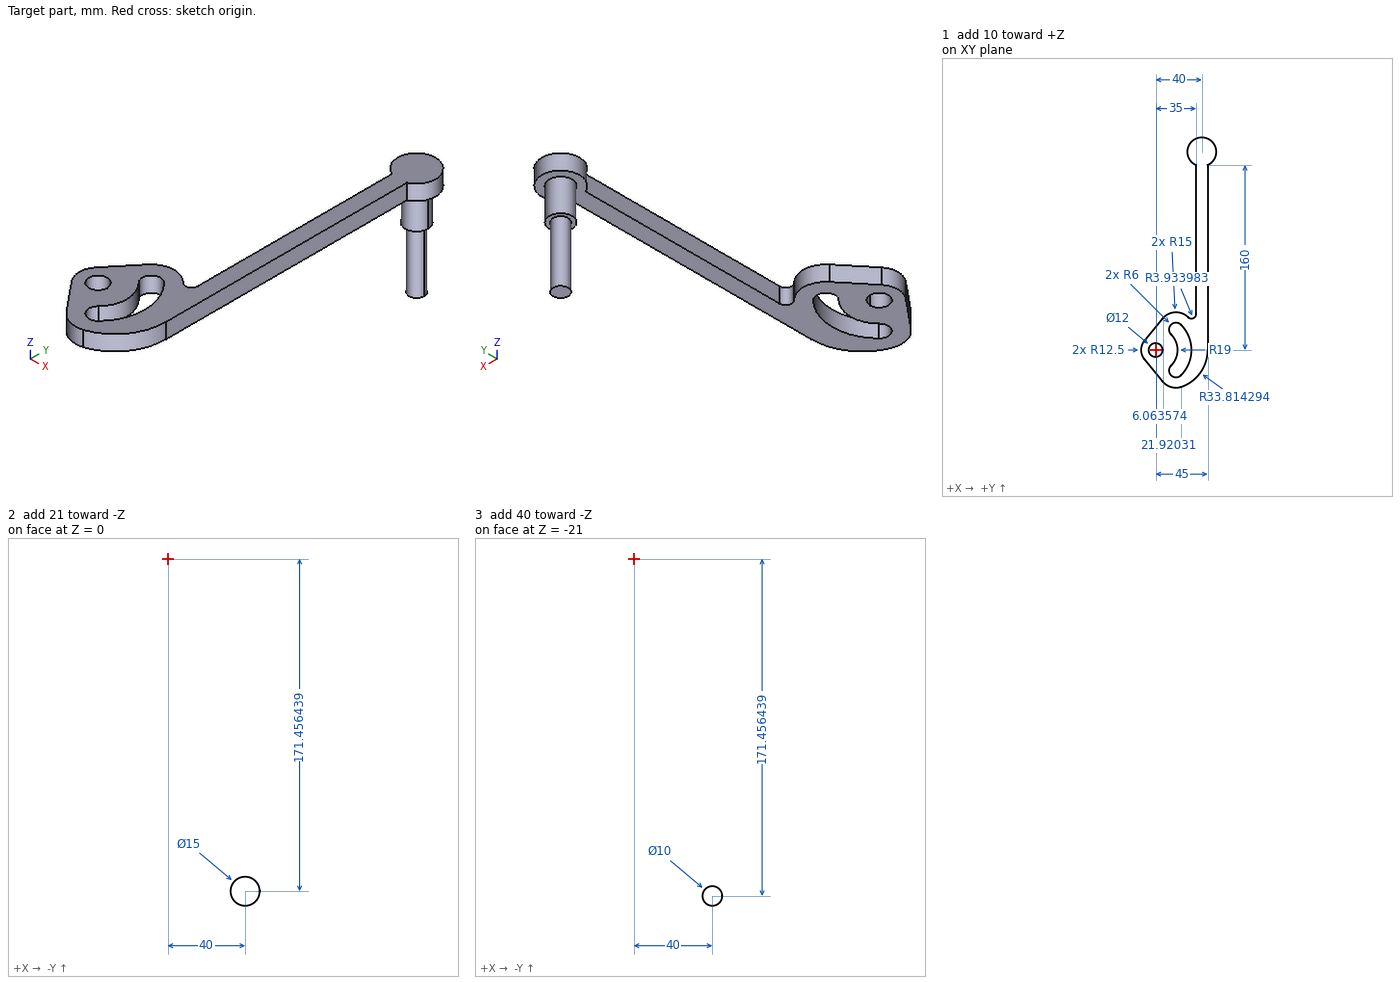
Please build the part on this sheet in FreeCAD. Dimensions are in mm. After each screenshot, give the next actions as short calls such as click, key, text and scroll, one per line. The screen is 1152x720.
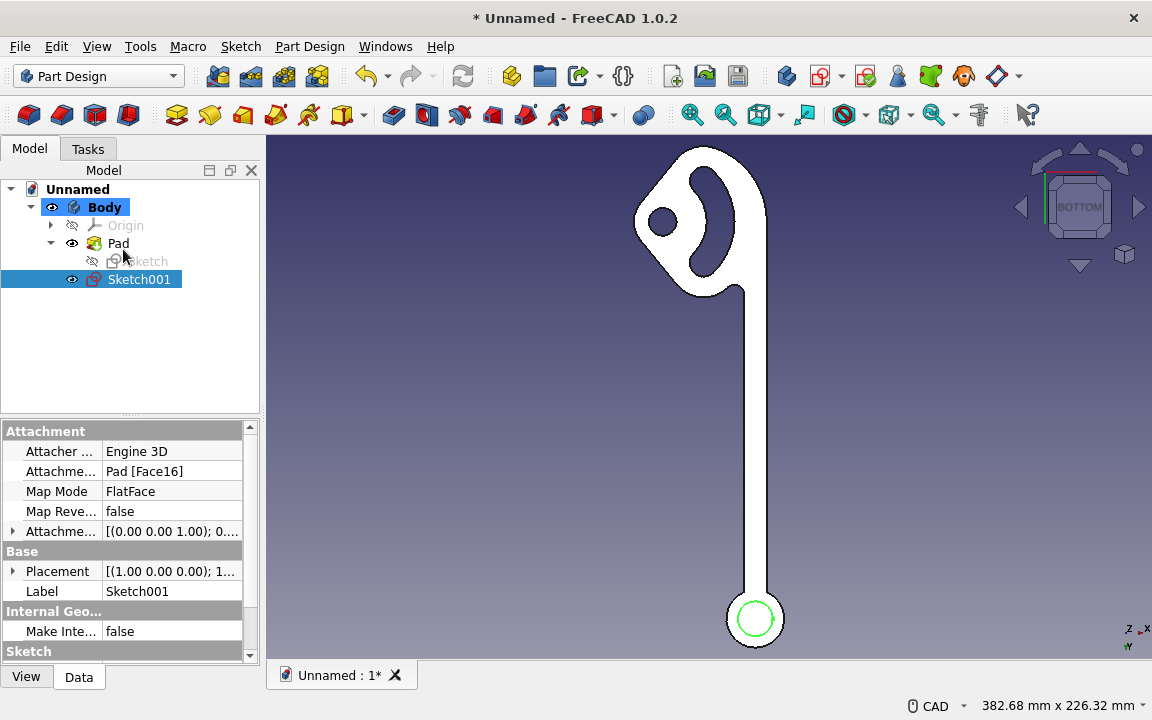
click(177, 116)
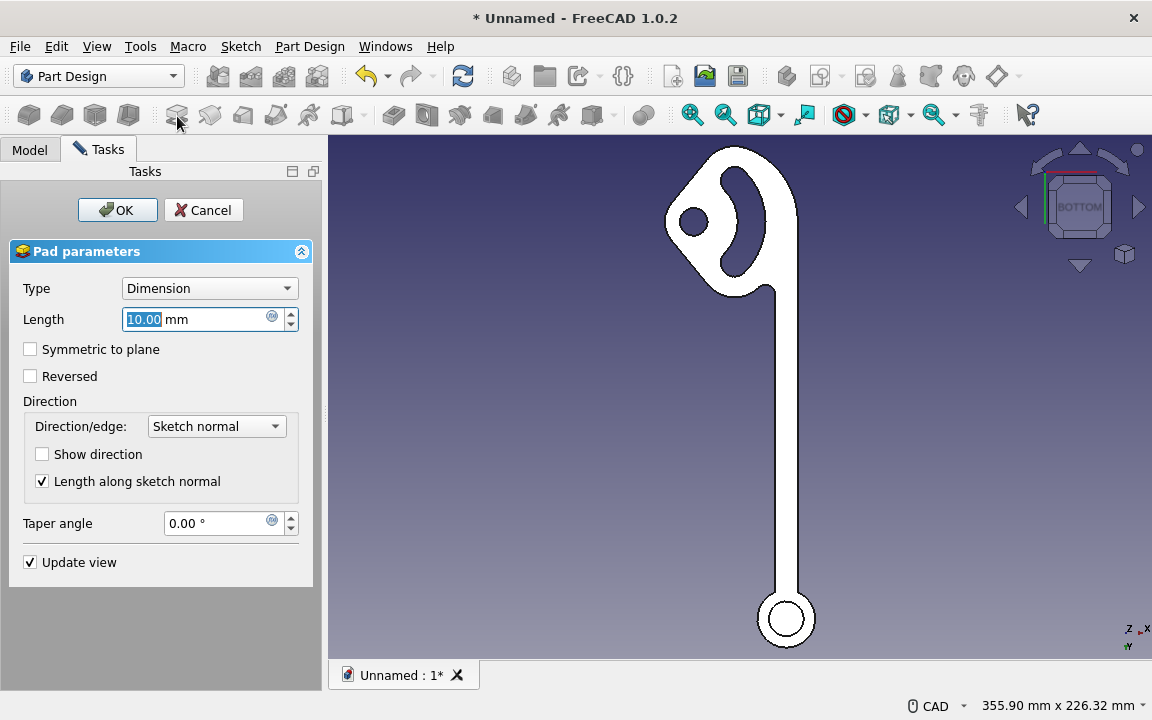
text(21)
key(Tab)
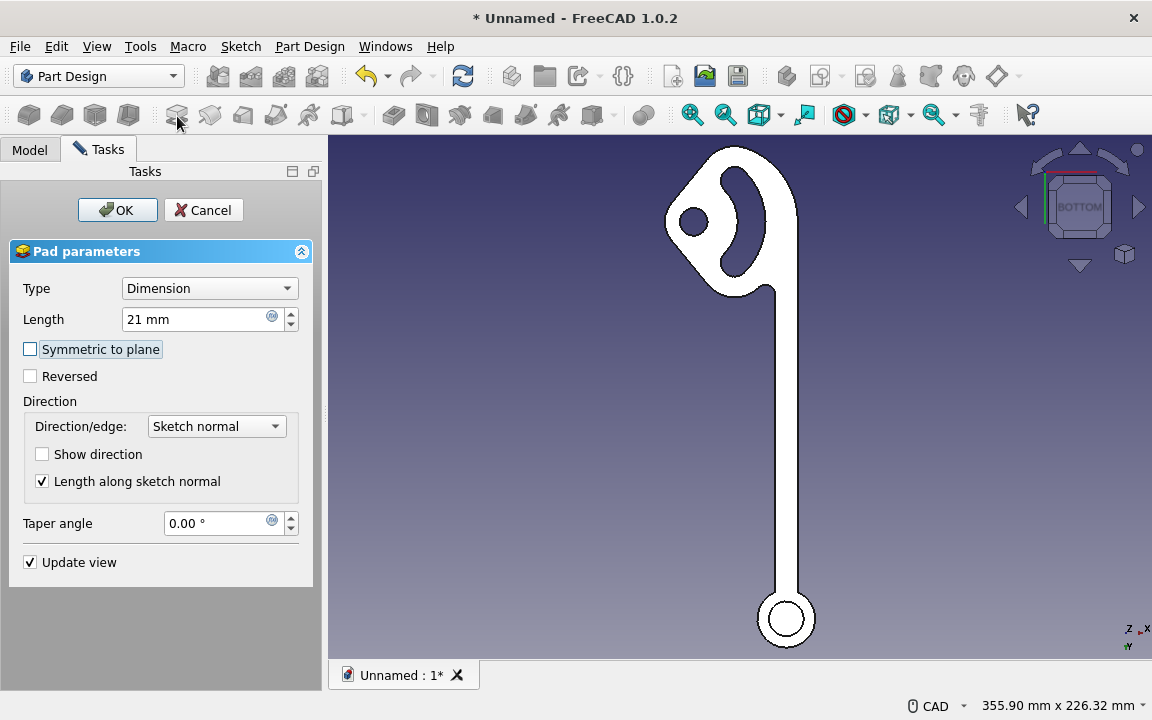
click(118, 210)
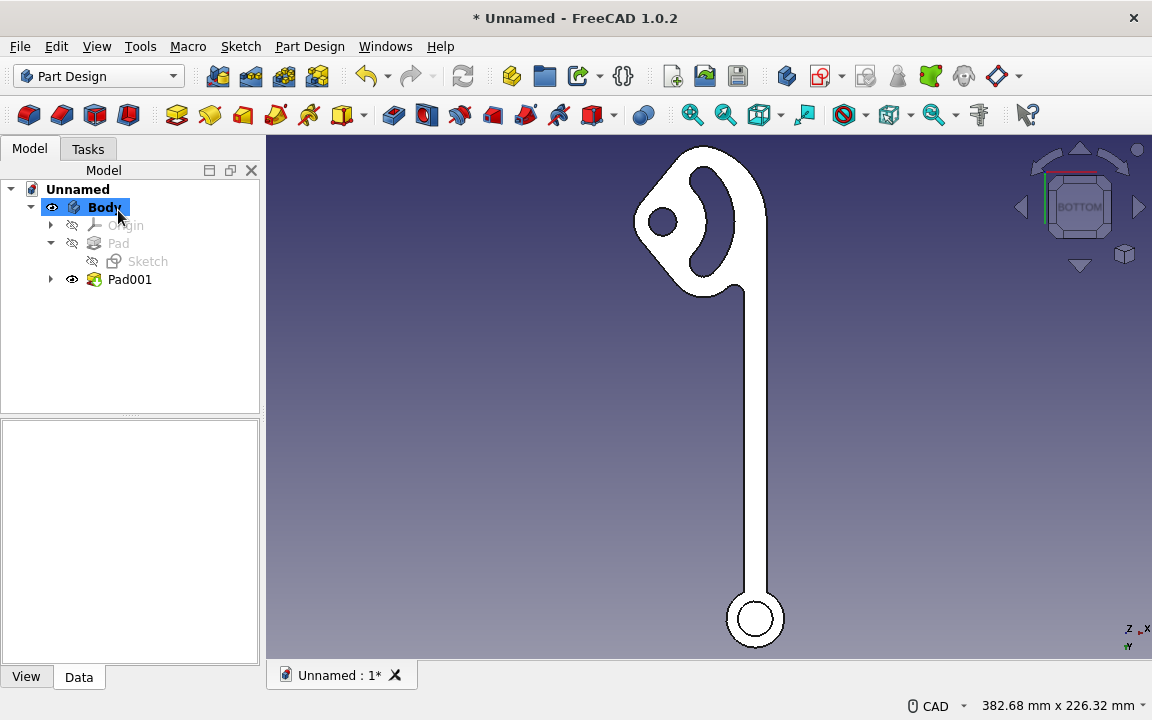
click(755, 618)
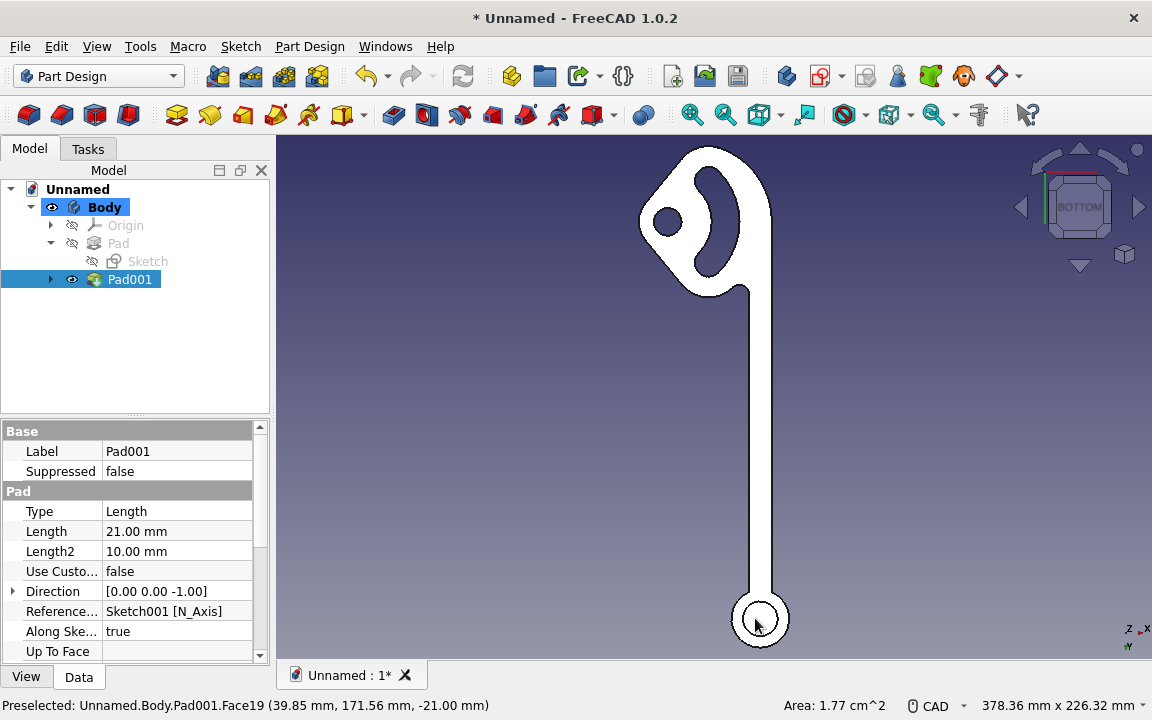
click(820, 76)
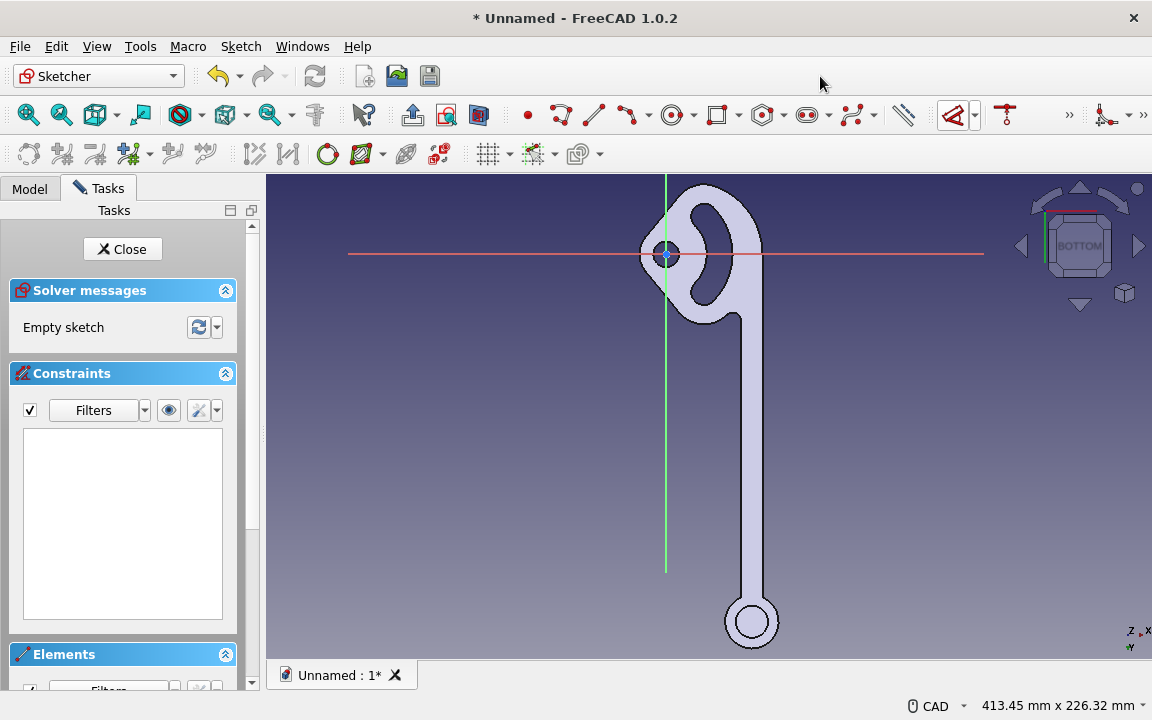
scroll(640, 416, down, 5)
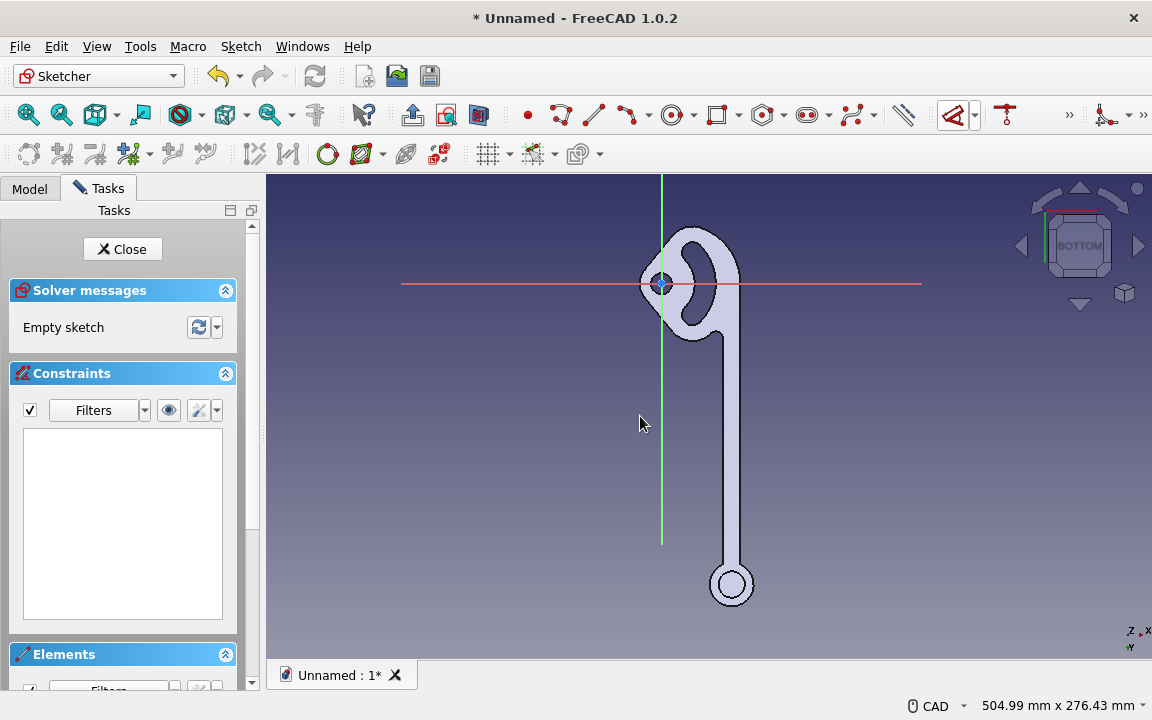
scroll(684, 496, up, 15)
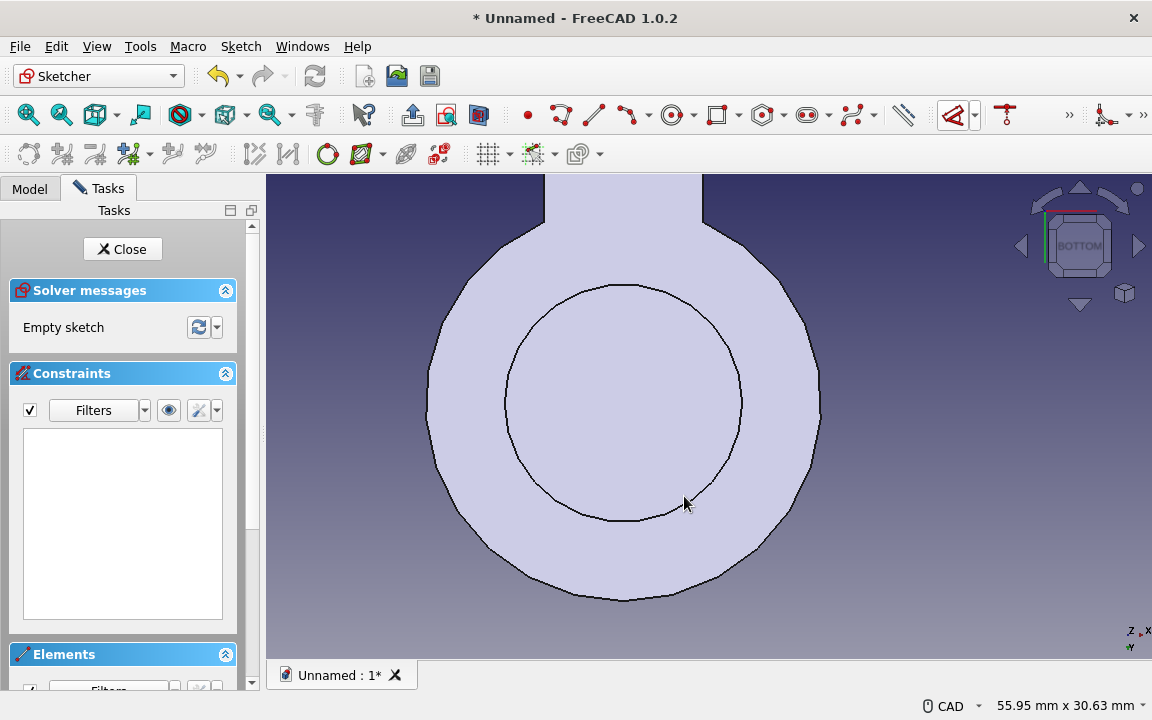
scroll(603, 387, up, 3)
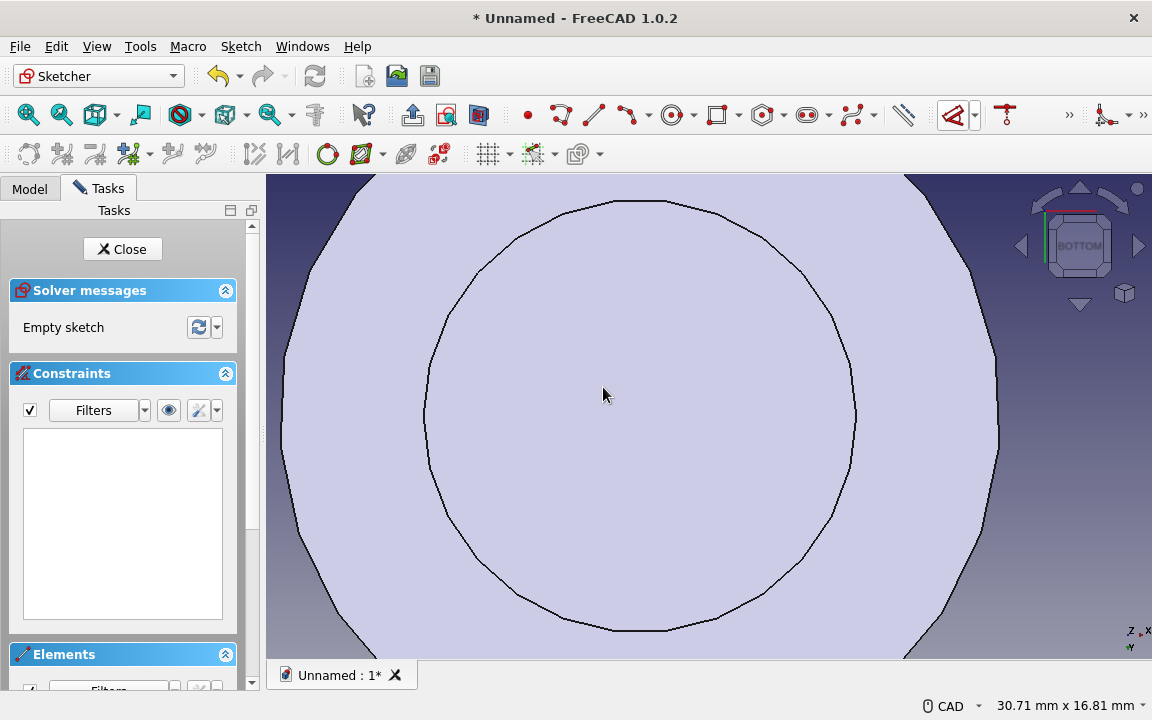
key(g)
key(c)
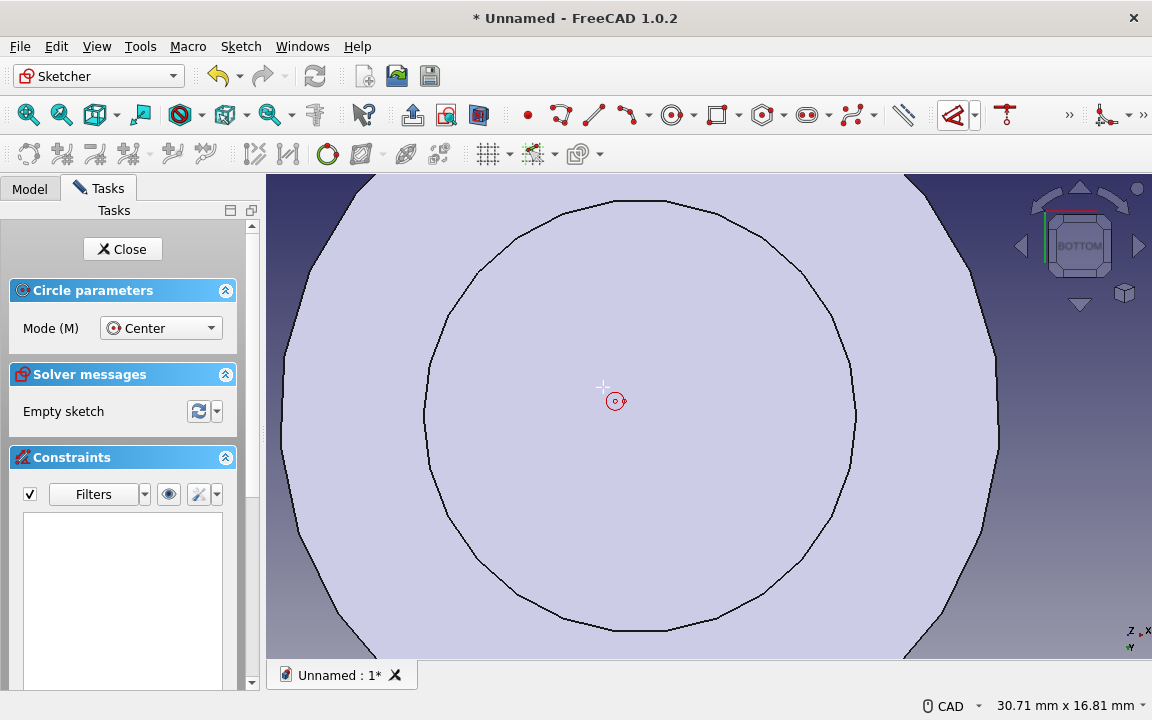
click(640, 416)
click(742, 314)
key(Escape)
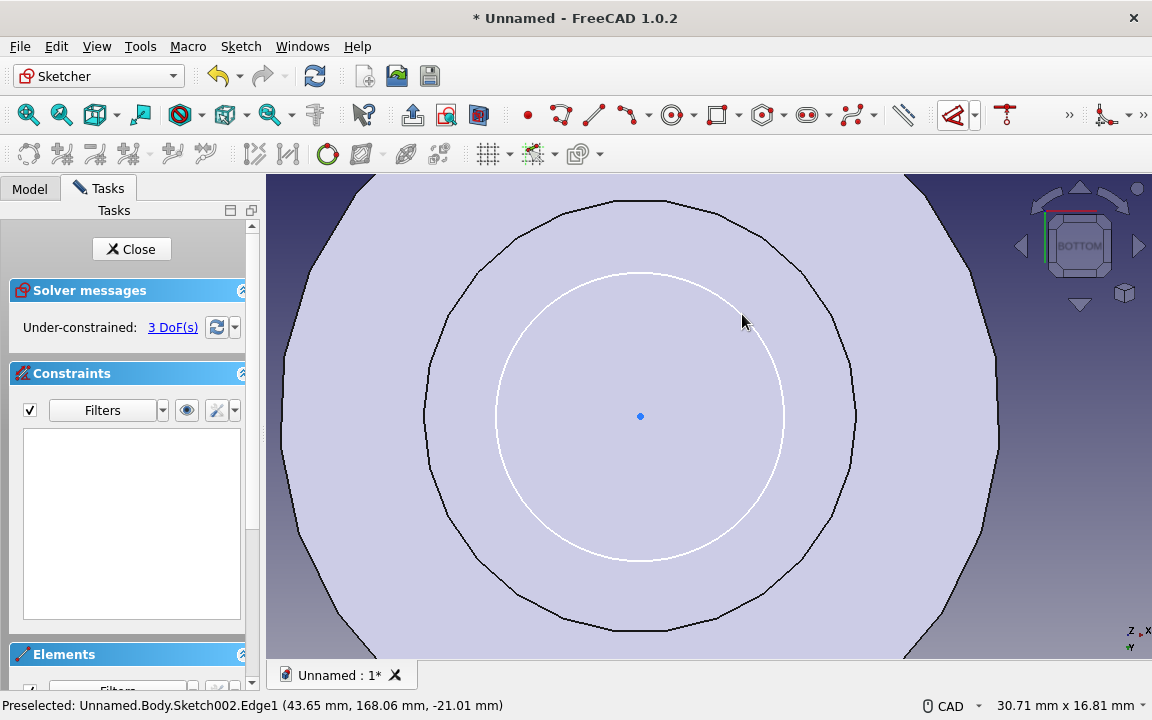
click(952, 116)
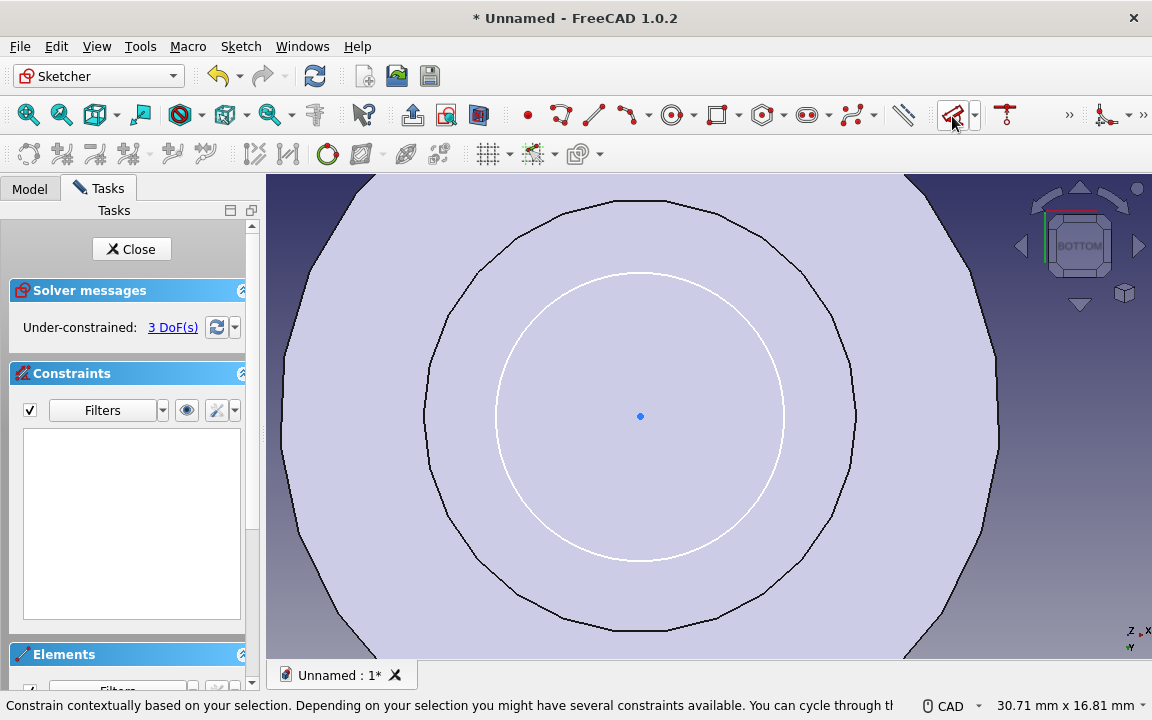
click(742, 315)
click(765, 292)